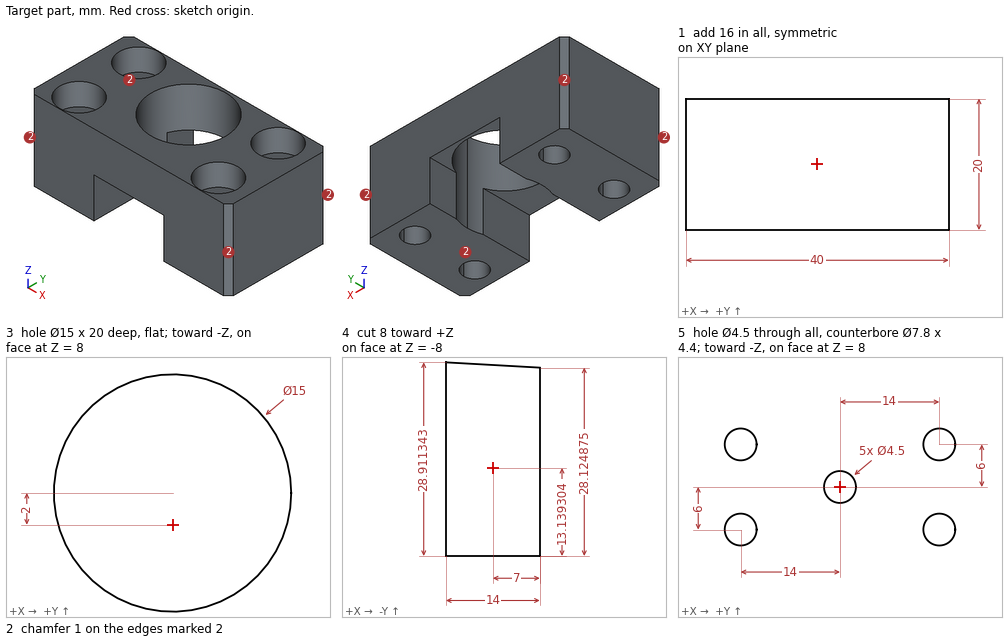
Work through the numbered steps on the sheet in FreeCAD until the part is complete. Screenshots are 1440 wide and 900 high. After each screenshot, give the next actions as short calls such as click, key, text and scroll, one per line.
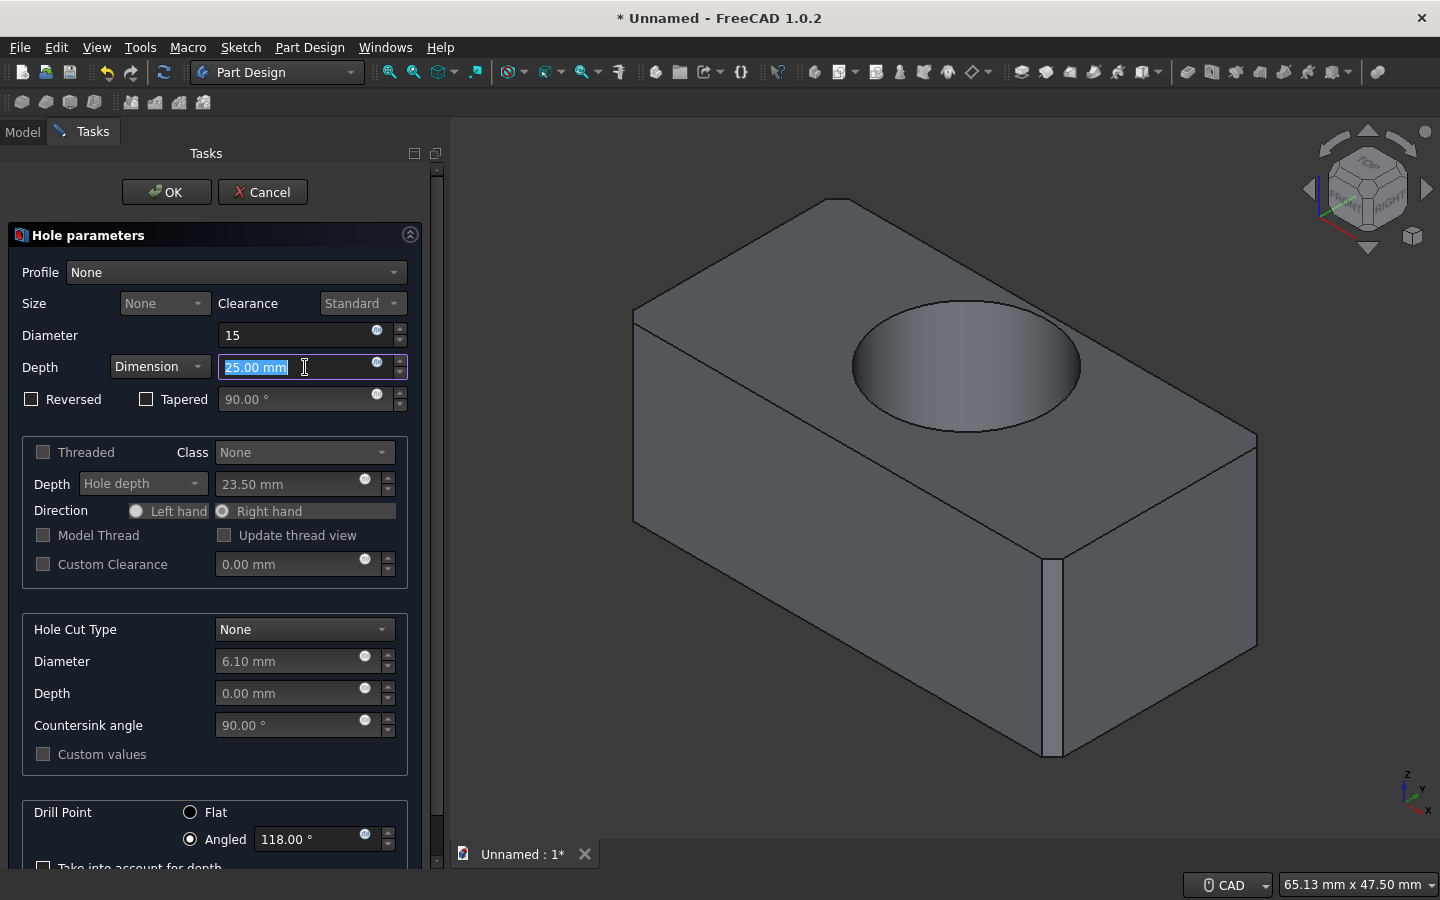
text(20)
key(Tab)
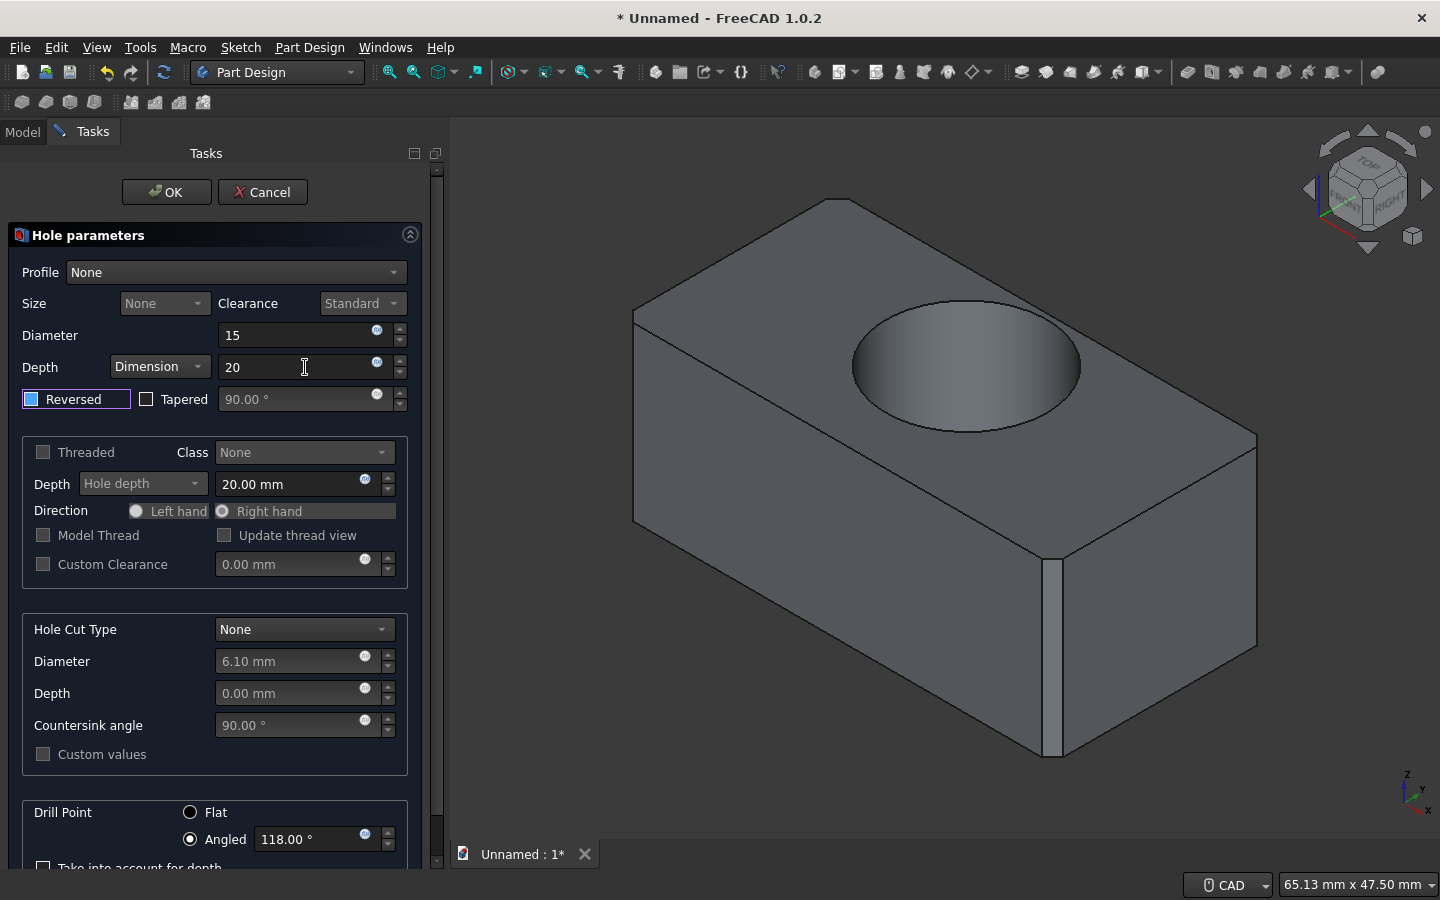
click(191, 812)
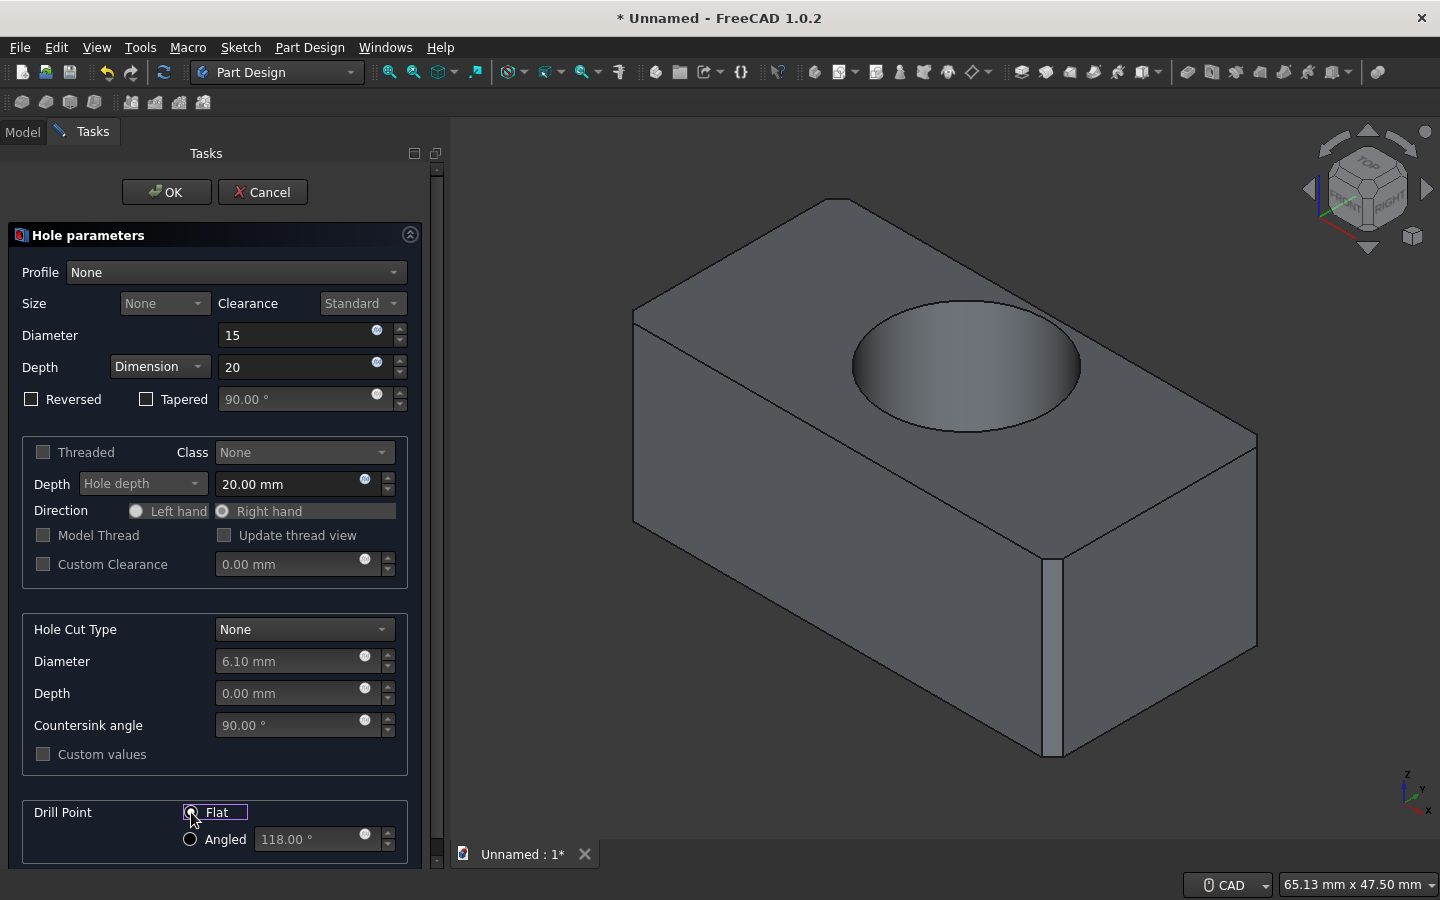
click(167, 192)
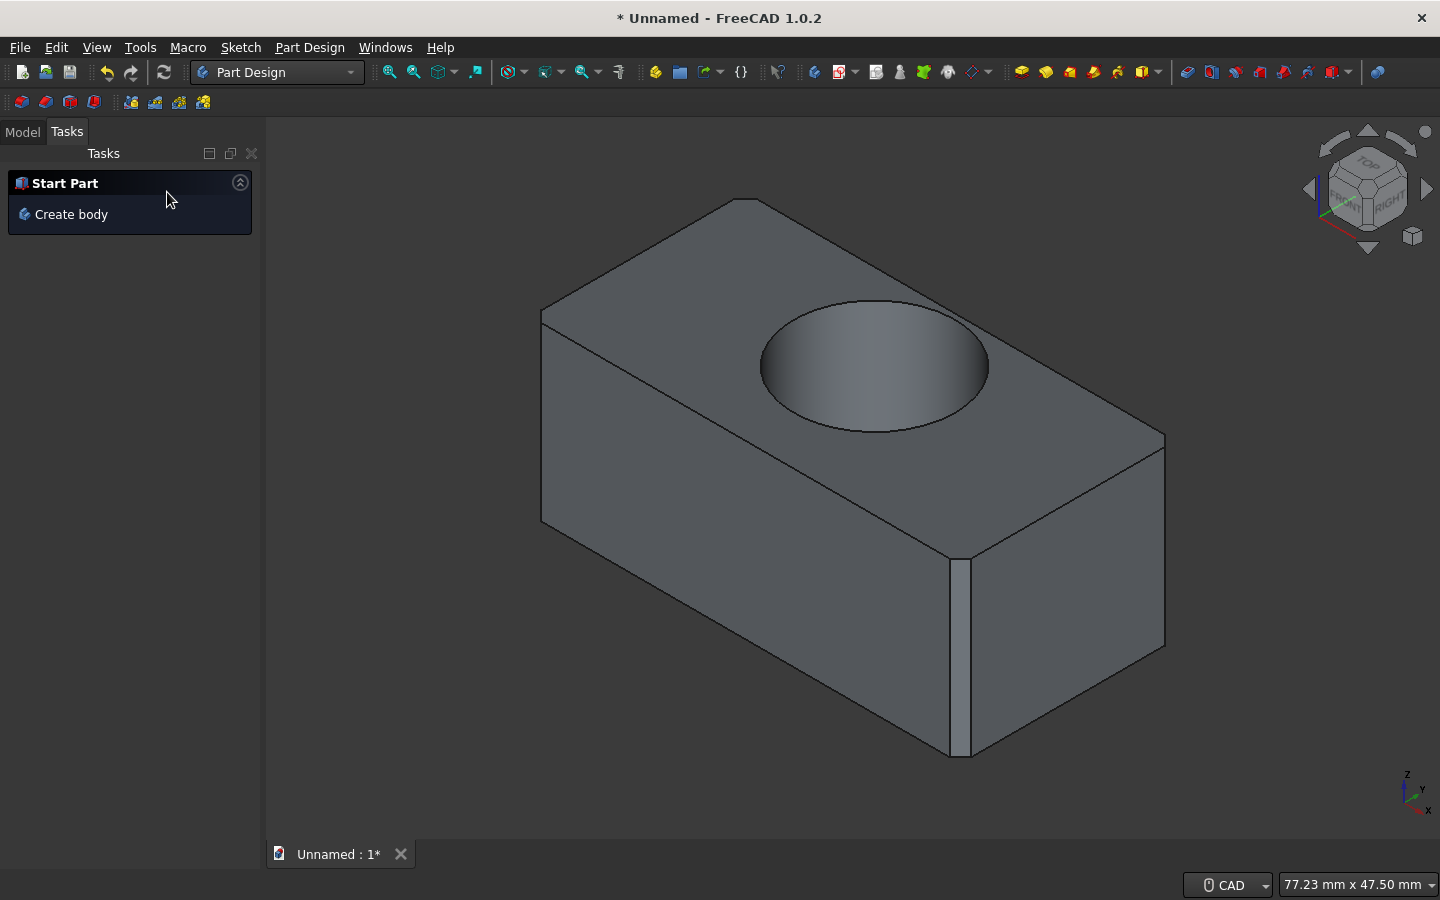
key(5)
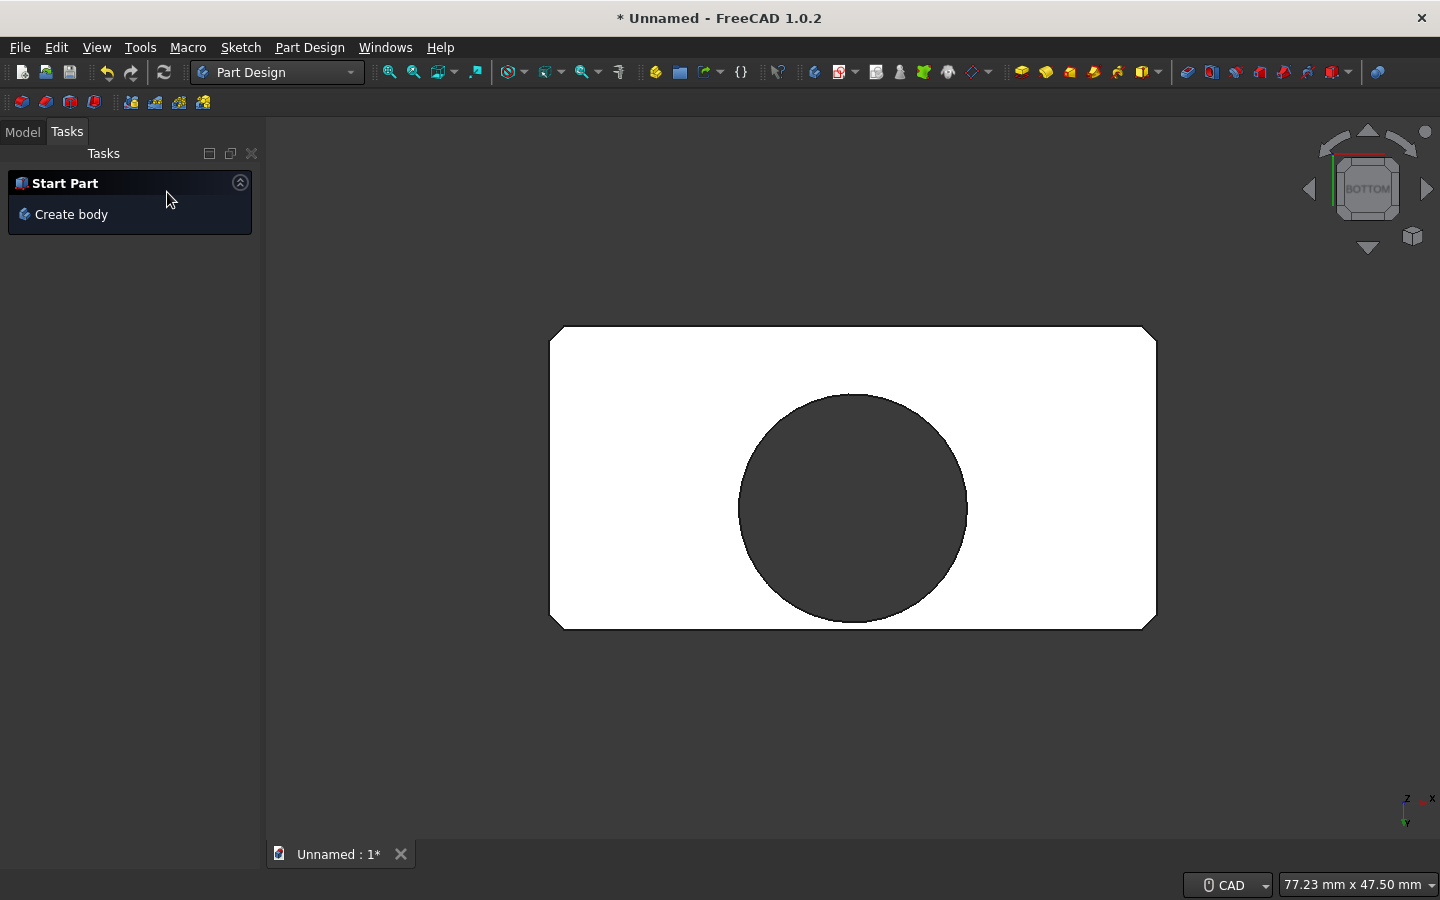
click(679, 434)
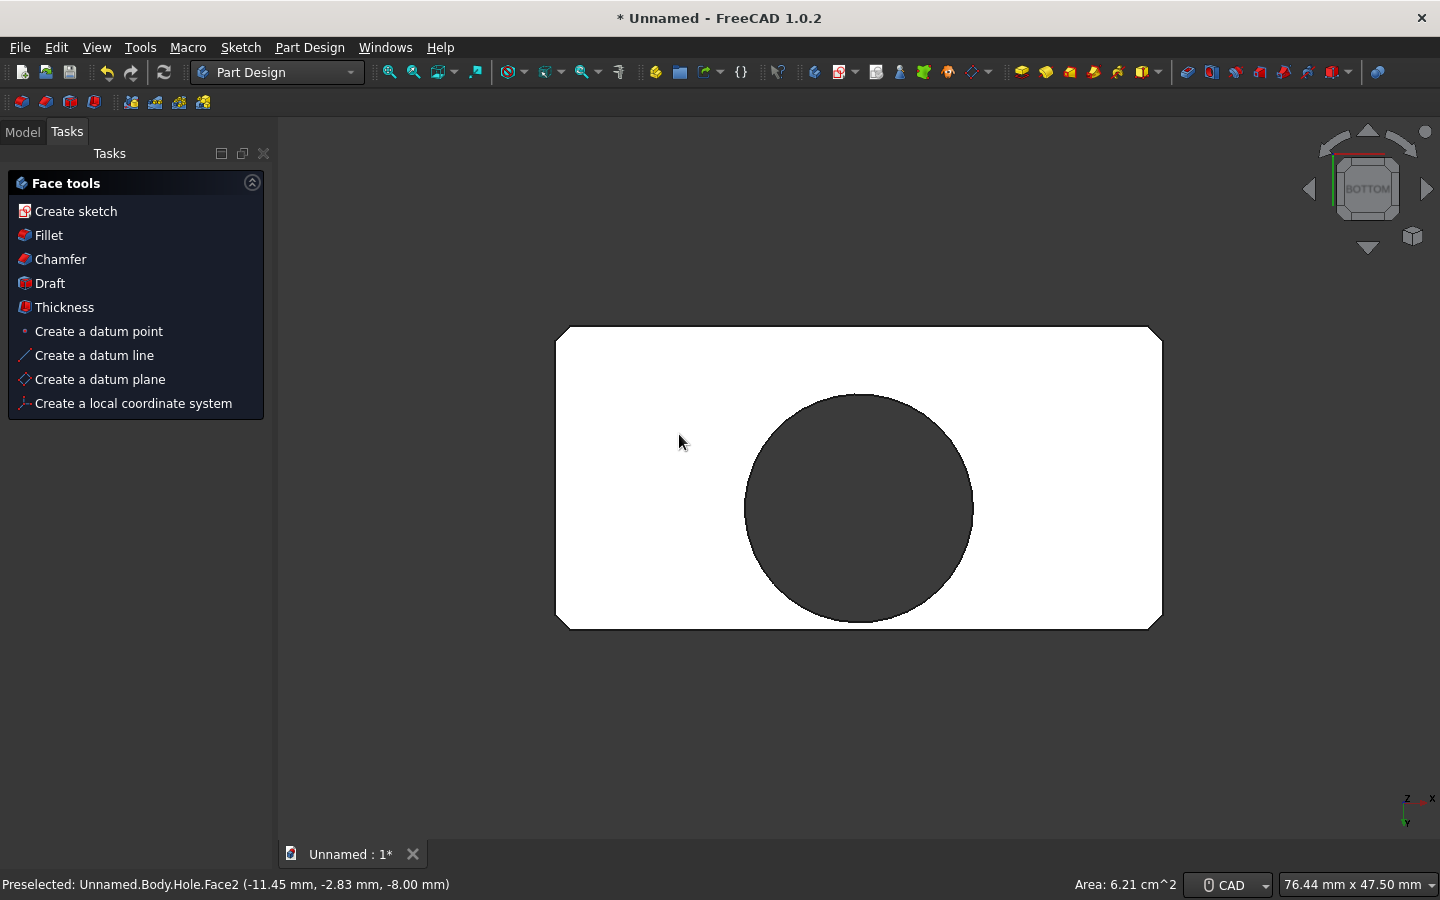
click(840, 72)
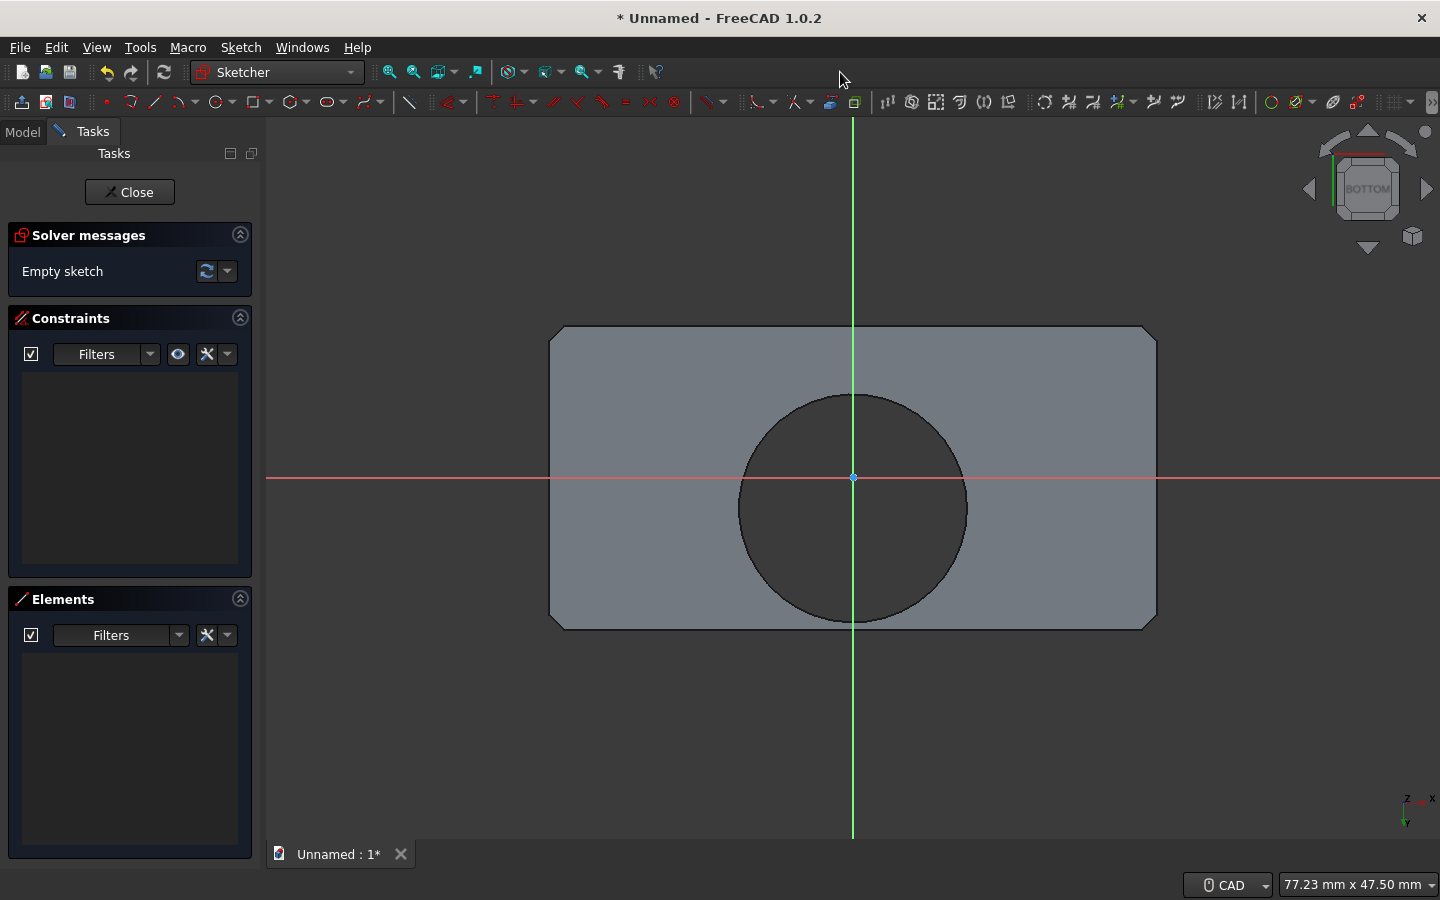
click(132, 102)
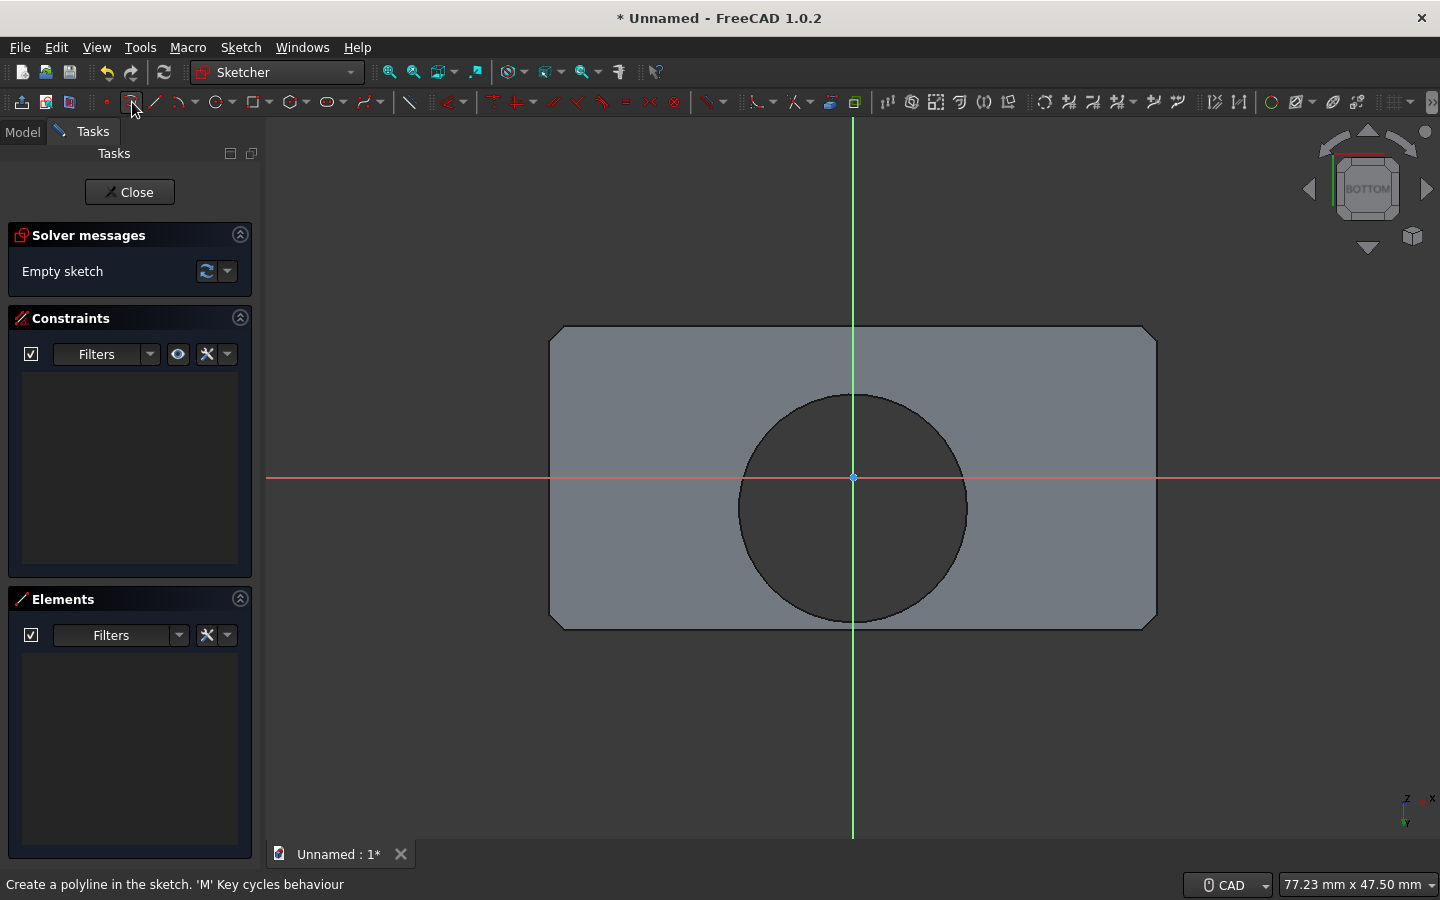
click(959, 678)
click(959, 250)
click(747, 238)
click(747, 678)
click(959, 679)
key(Escape)
key(Escape)